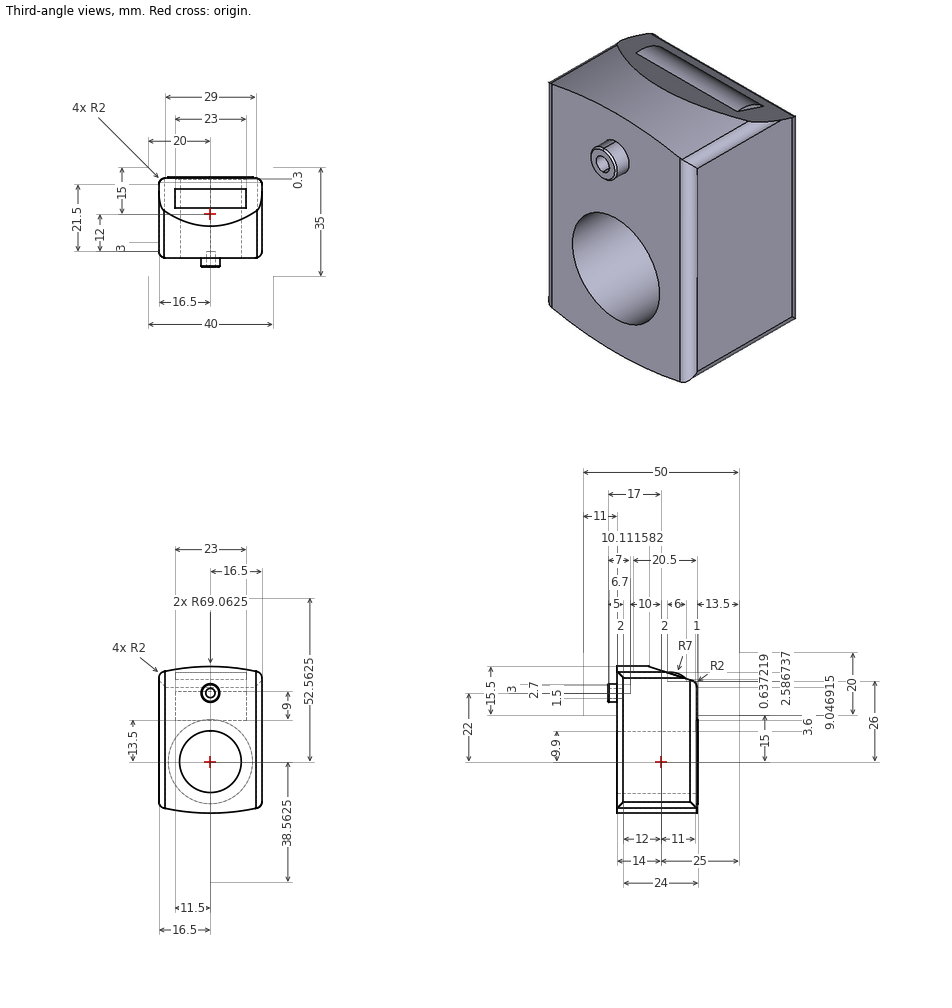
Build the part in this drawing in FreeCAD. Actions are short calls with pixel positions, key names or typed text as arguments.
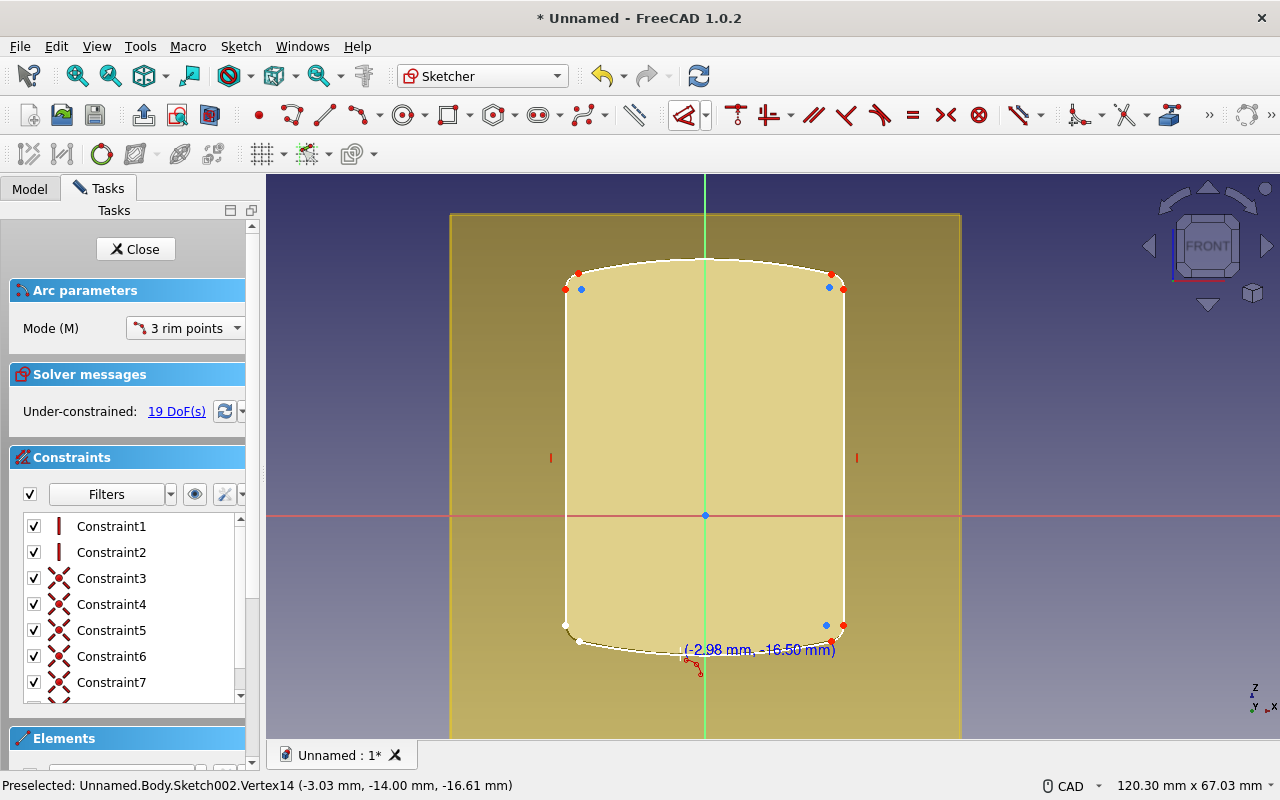
click(579, 642)
click(566, 626)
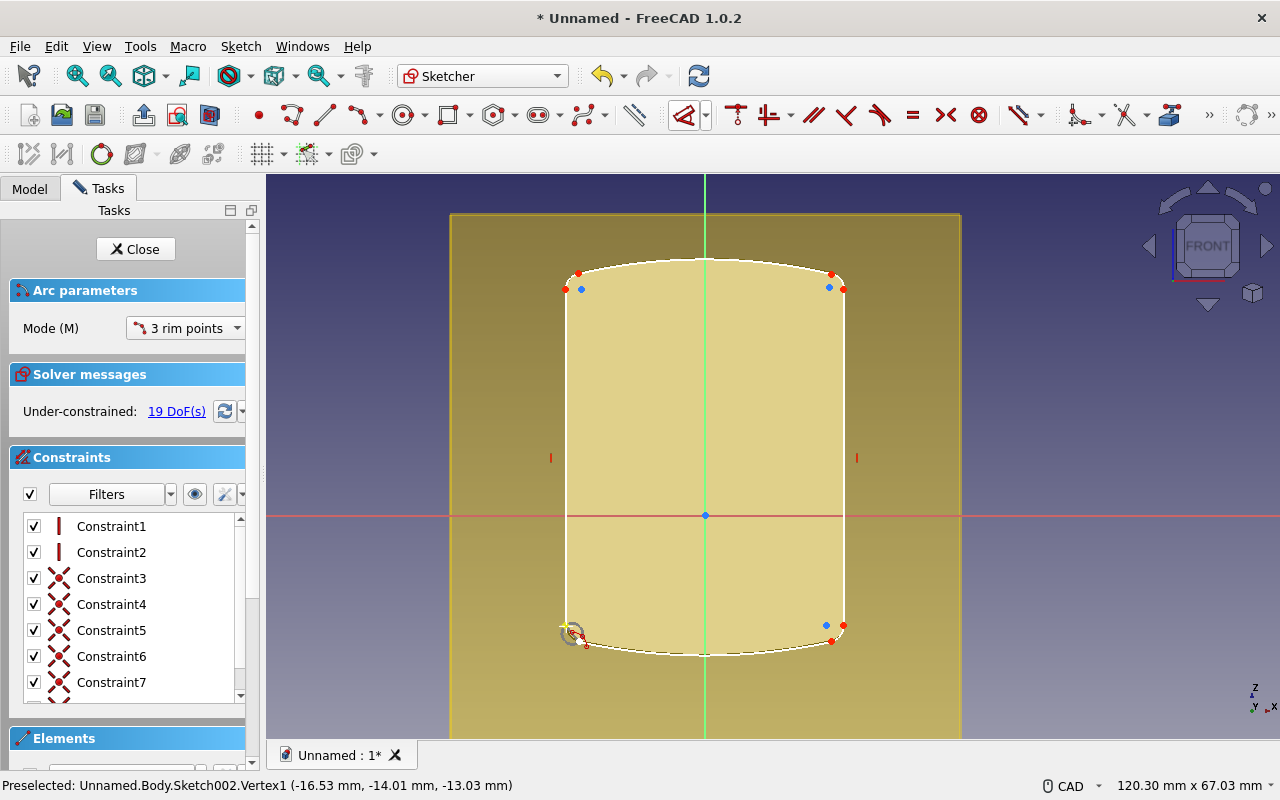
scroll(570, 635, up, 8)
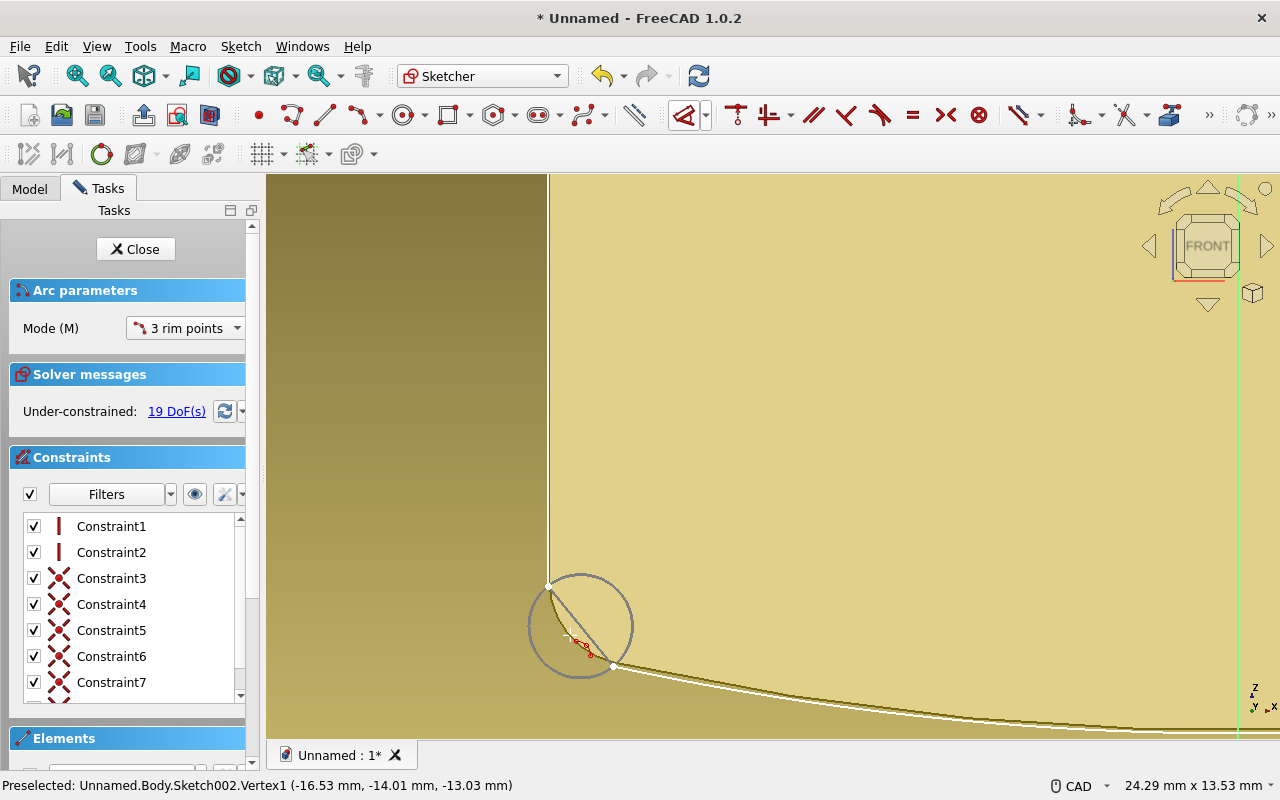
click(568, 633)
key(Escape)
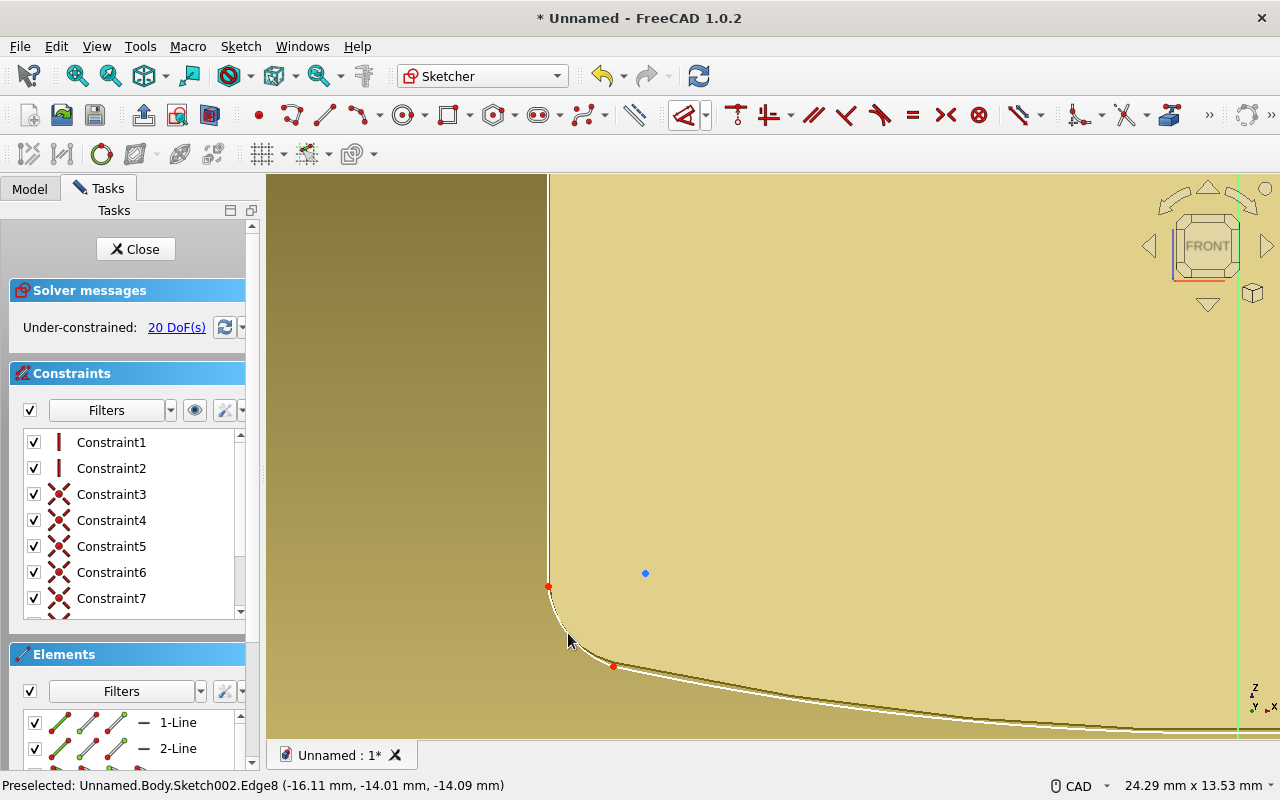
scroll(570, 635, down, 8)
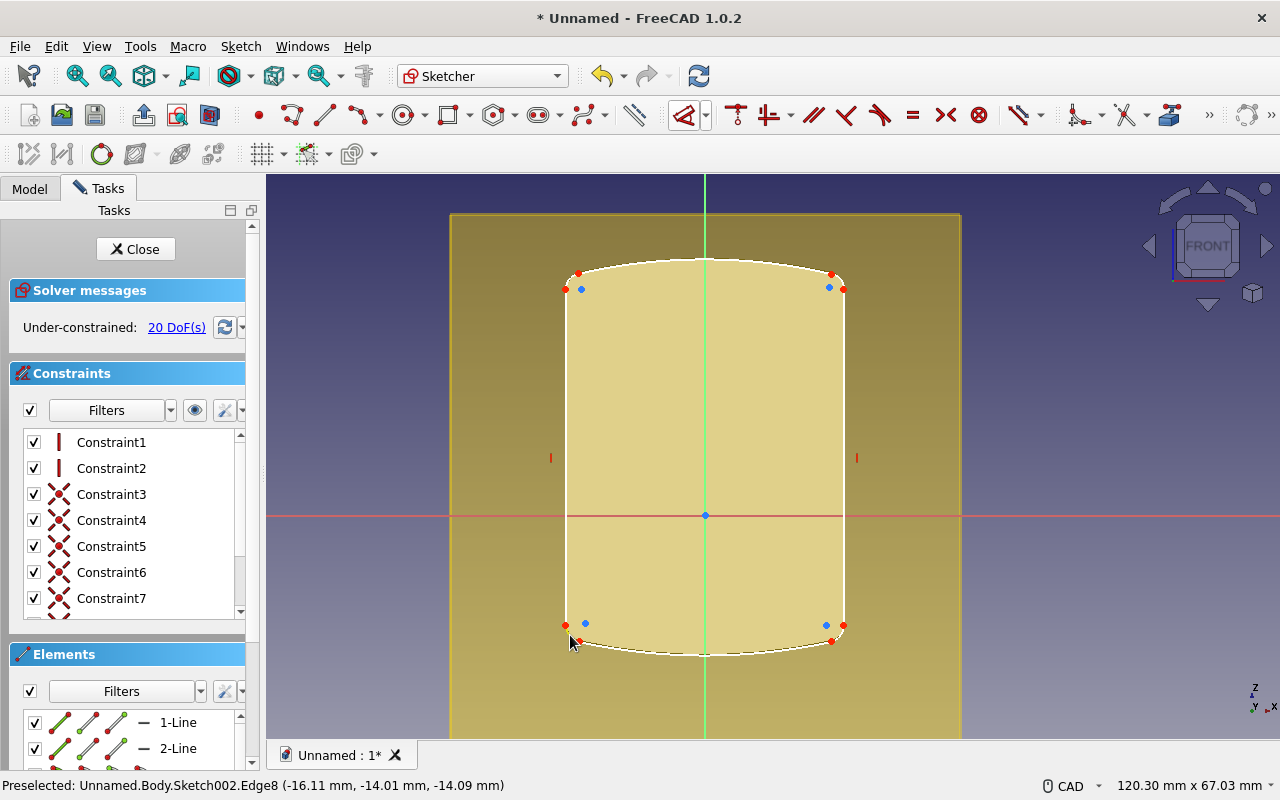
click(566, 559)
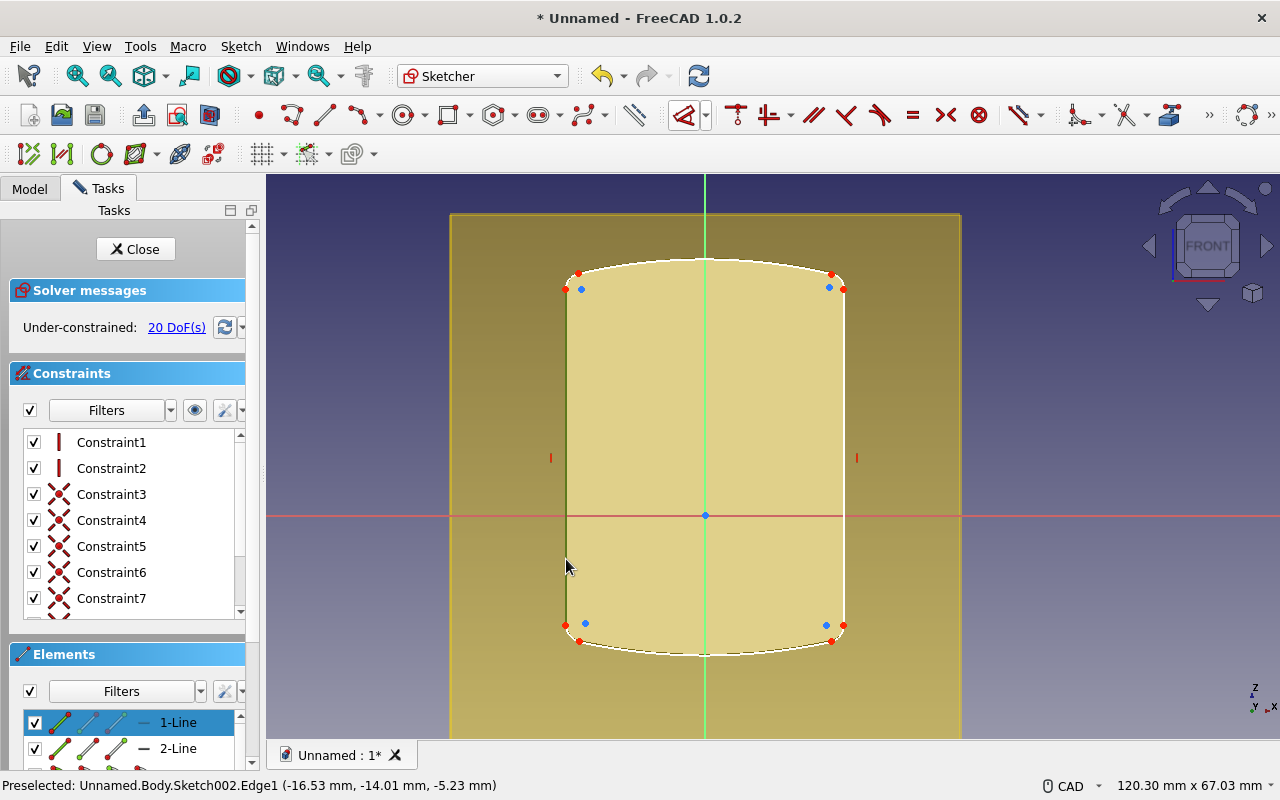
scroll(569, 279, up, 2)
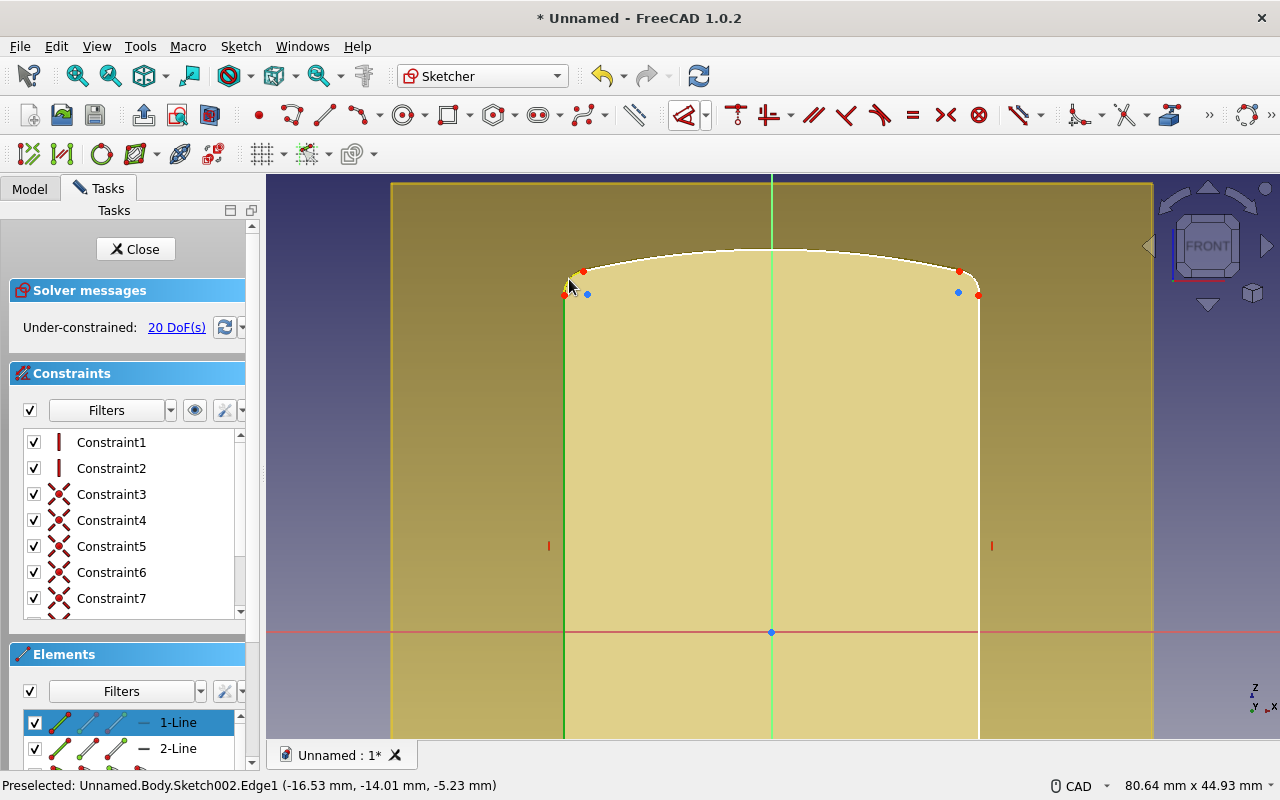
click(569, 279)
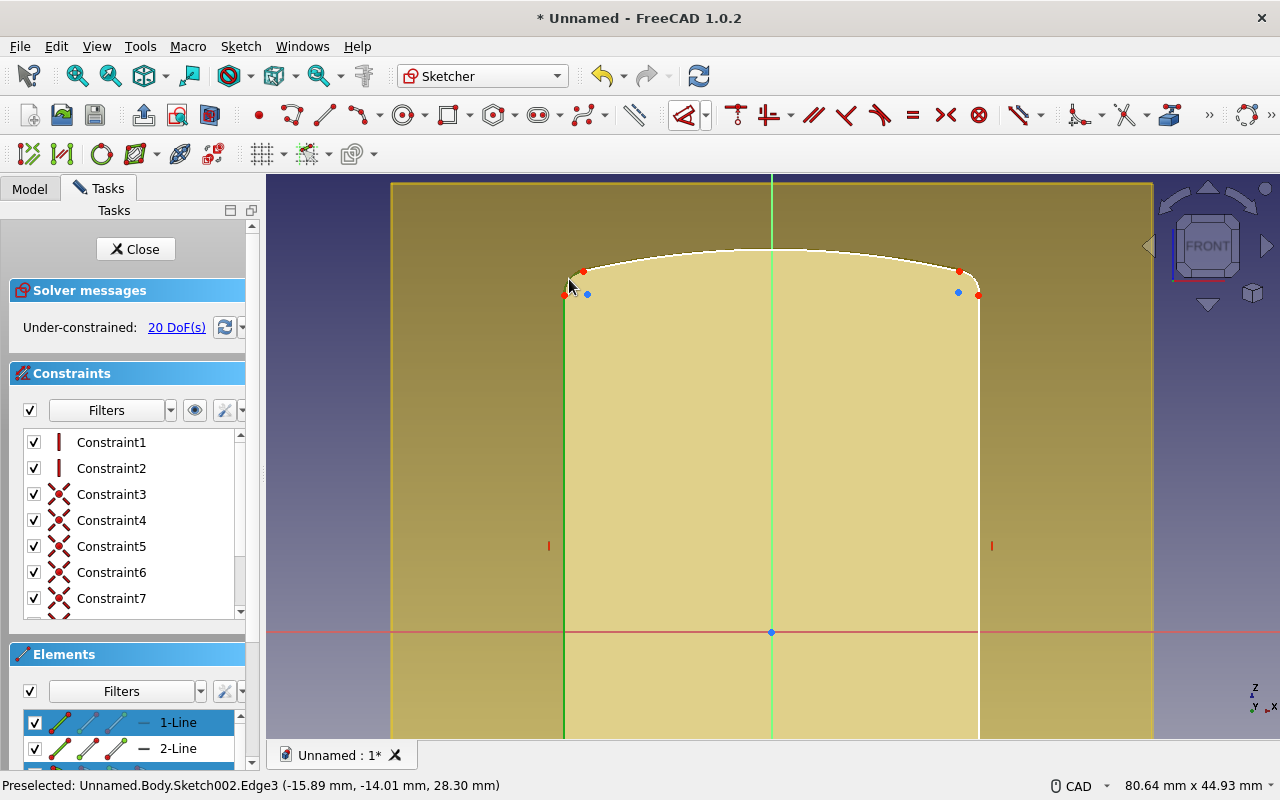
click(880, 116)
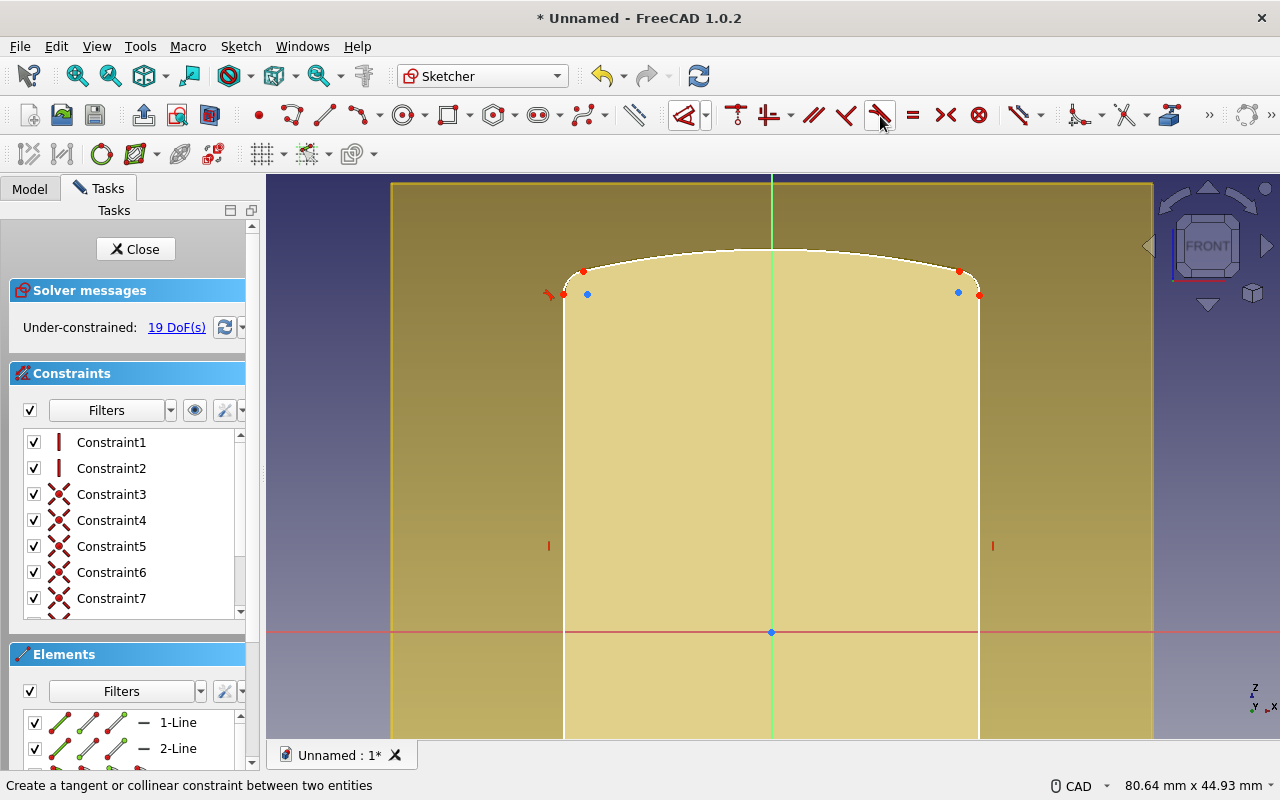
click(564, 646)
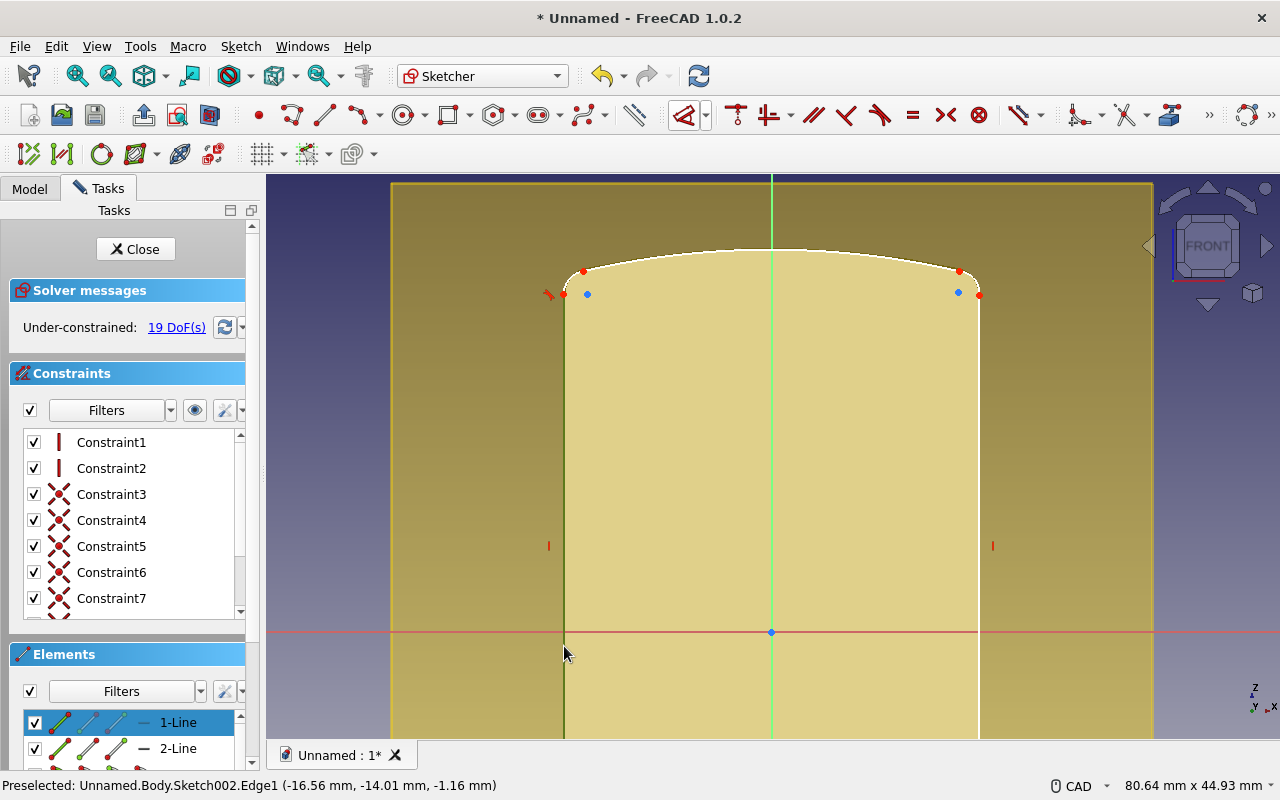
scroll(567, 278, down, 2)